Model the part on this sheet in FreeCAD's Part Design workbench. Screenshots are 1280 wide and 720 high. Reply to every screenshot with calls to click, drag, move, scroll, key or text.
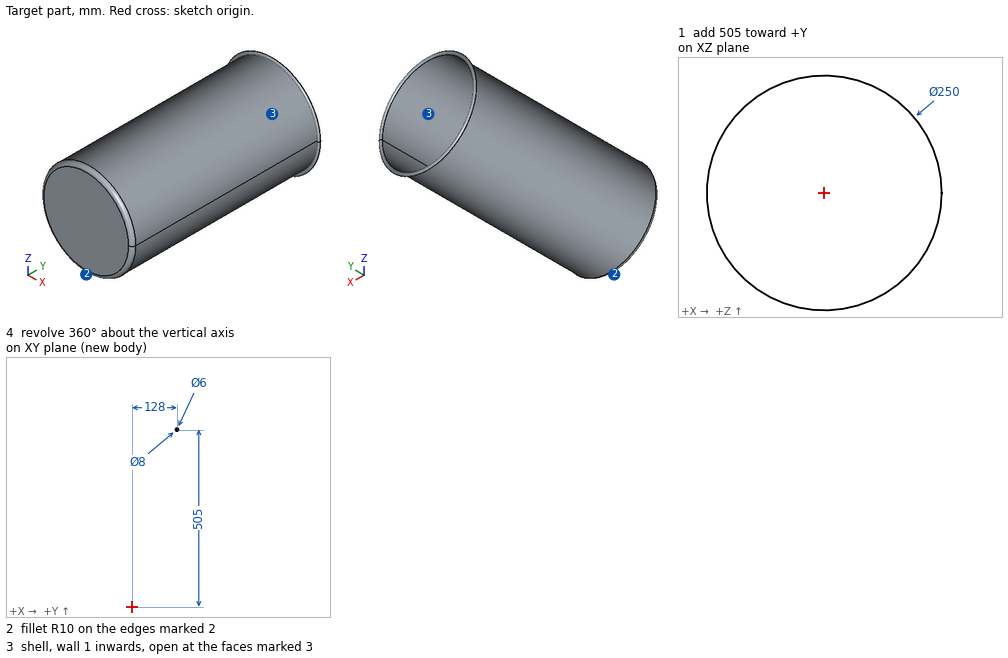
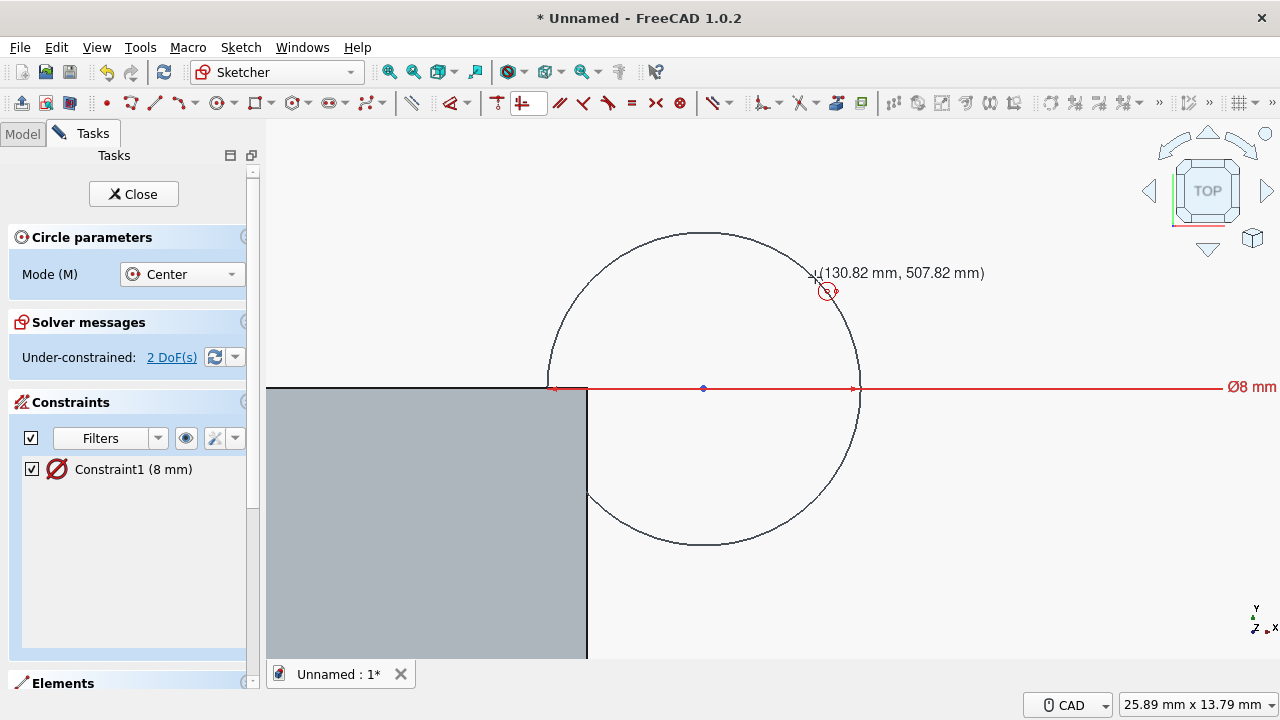
click(704, 389)
move(788, 305)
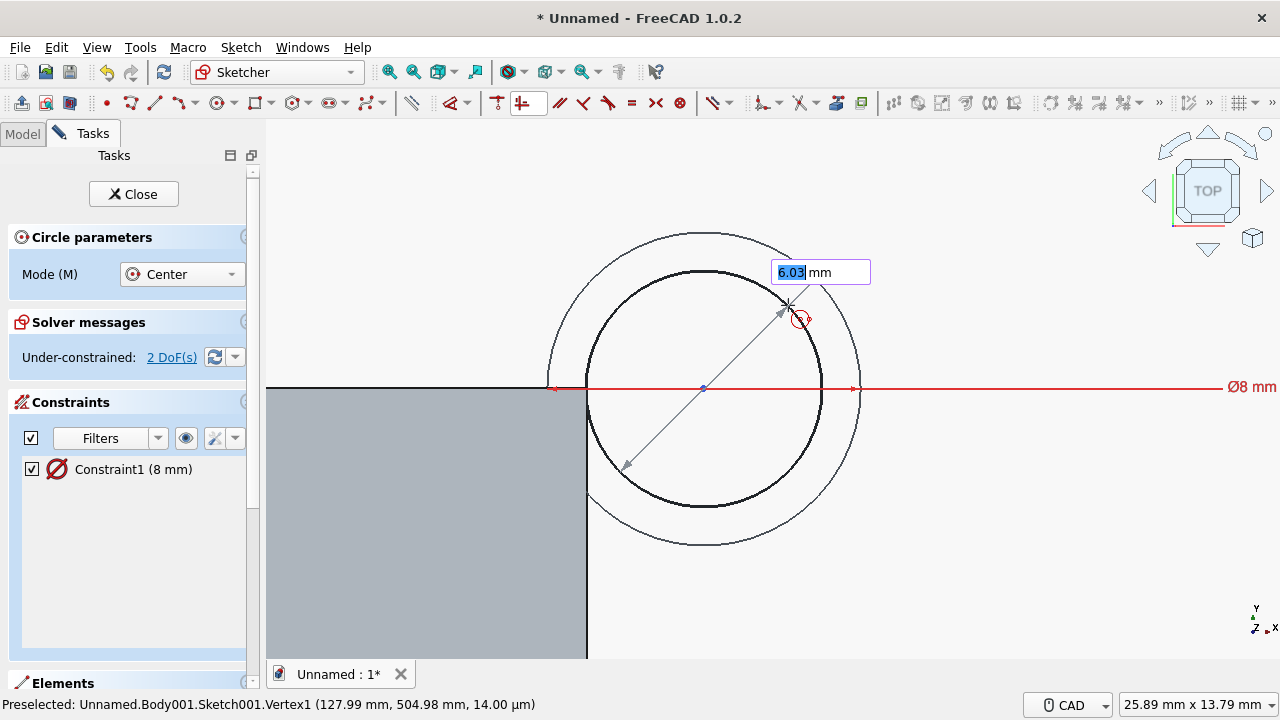
text(6)
key(Return)
key(Escape)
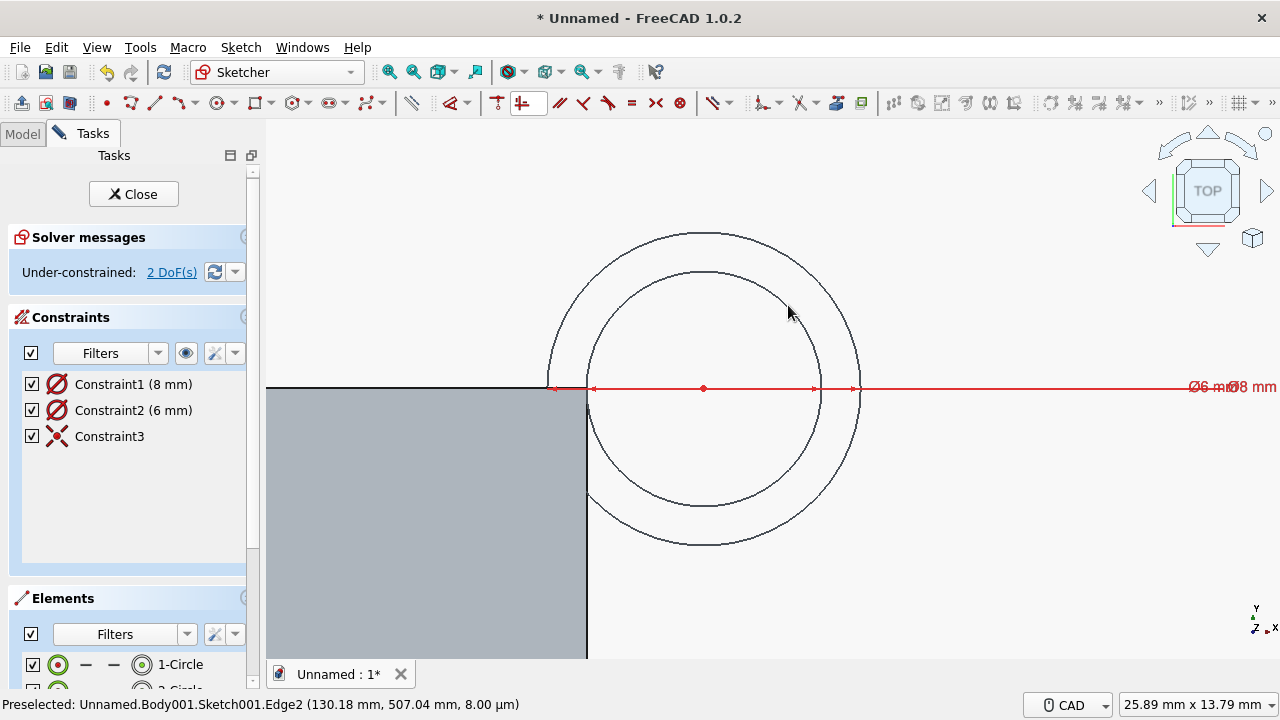
key(d)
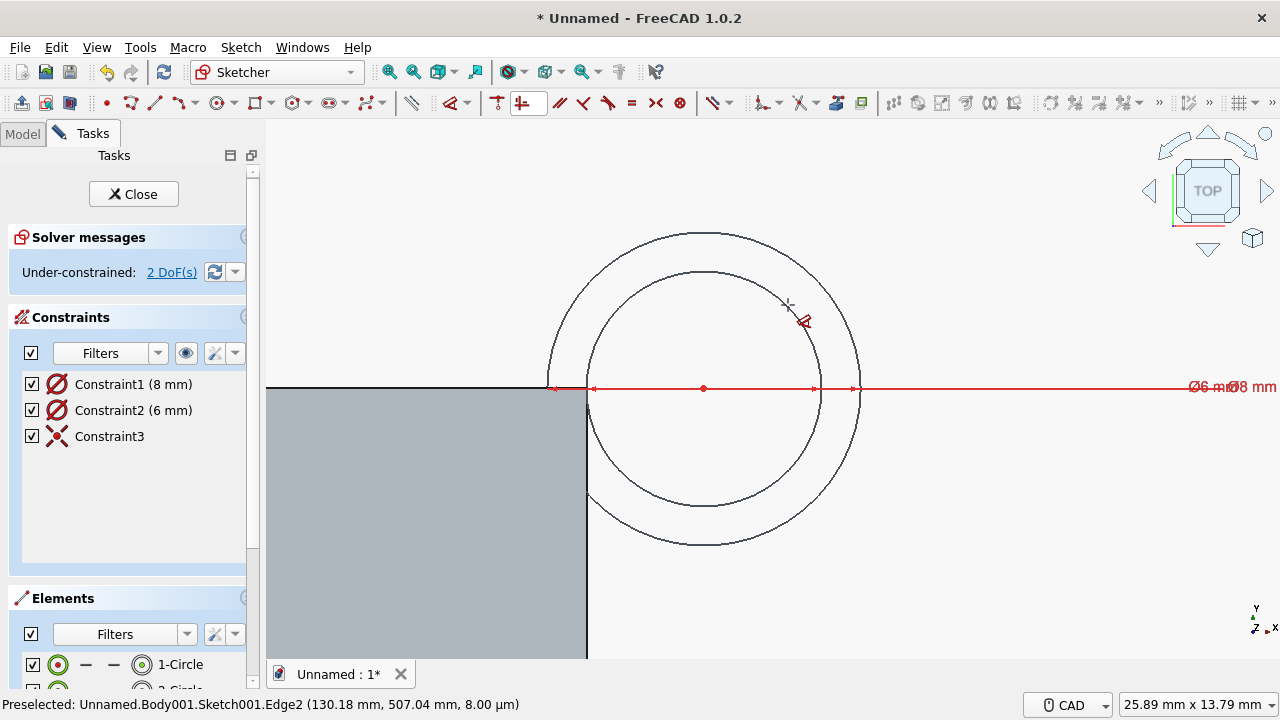
click(704, 389)
click(499, 355)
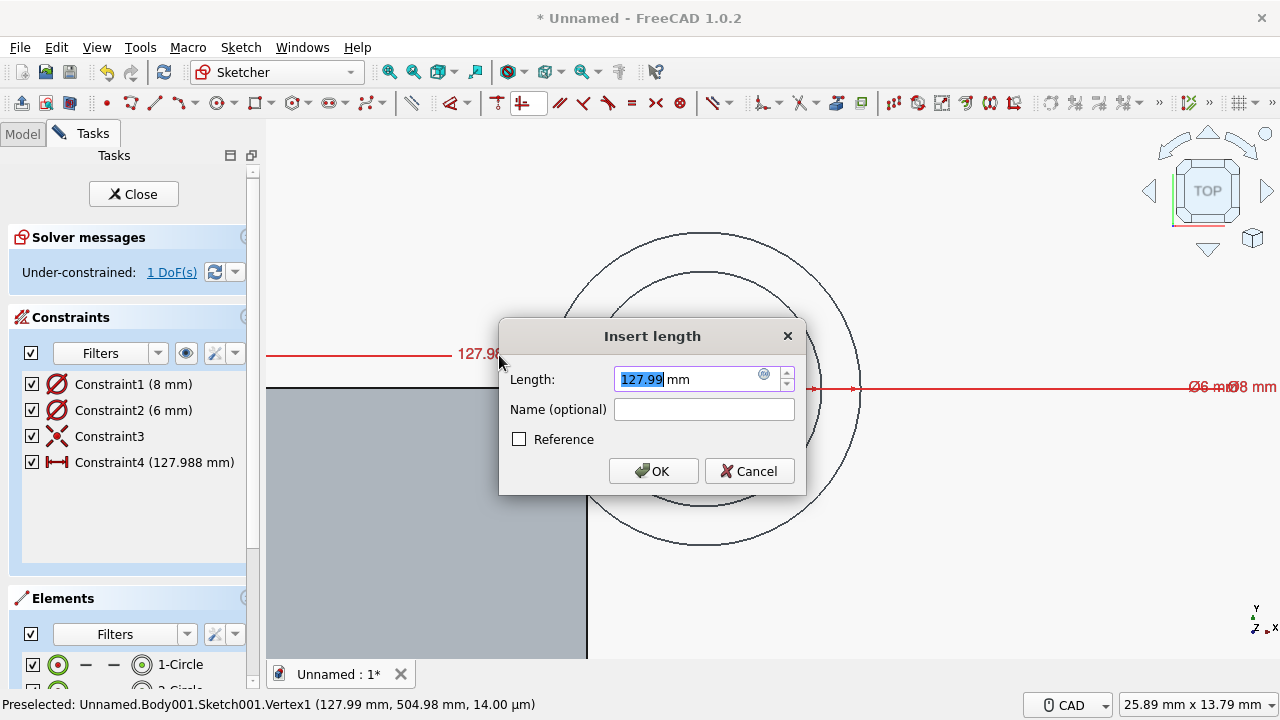
text(128)
key(Return)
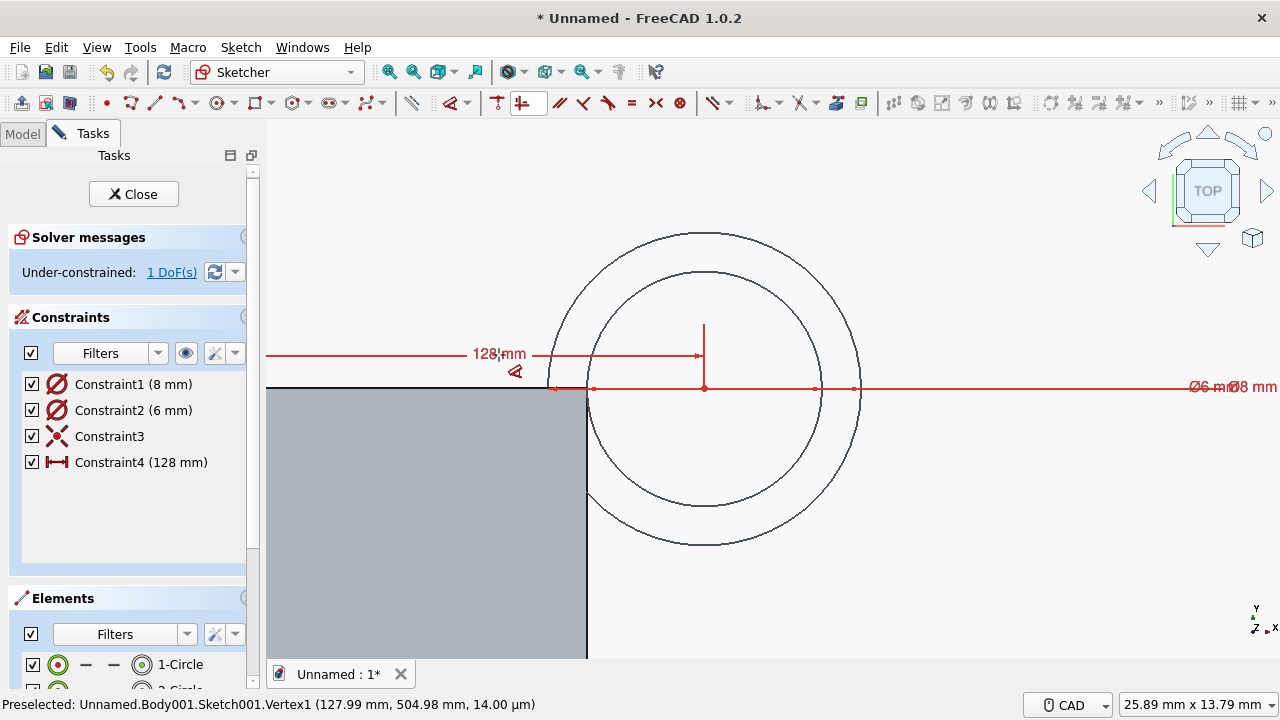
click(704, 389)
click(738, 454)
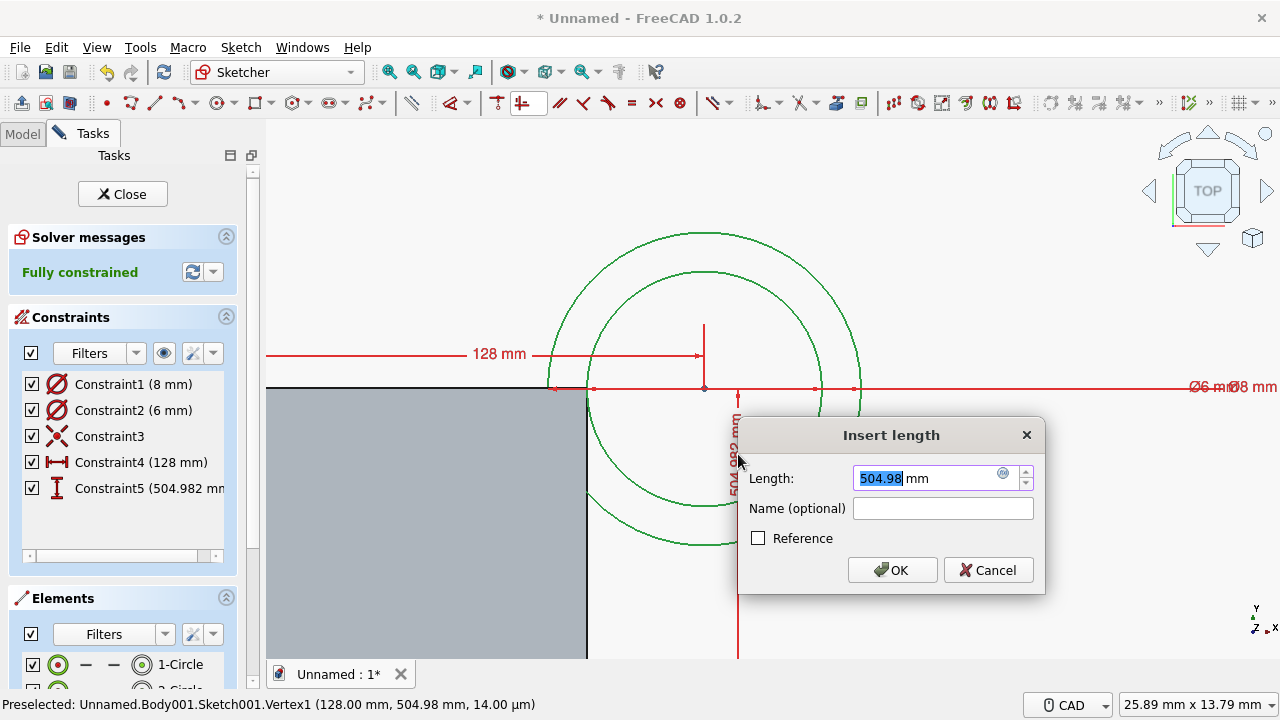
text(505)
key(Return)
key(Escape)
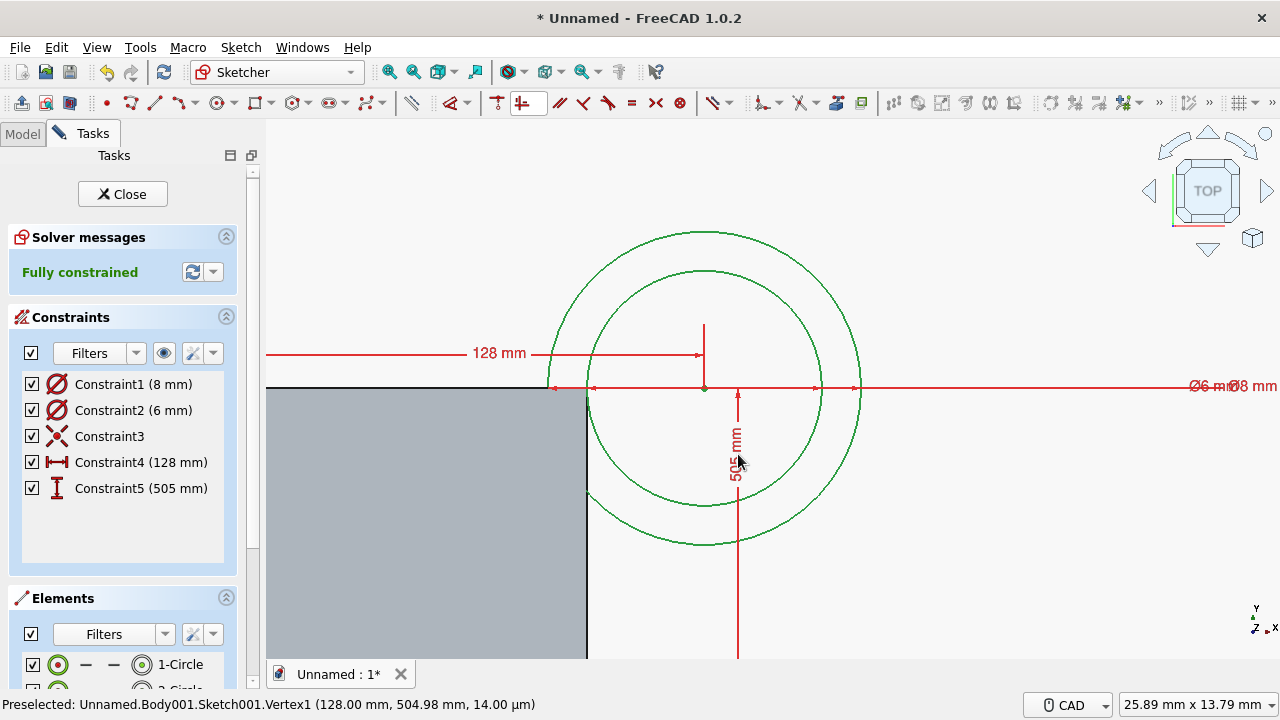
click(123, 194)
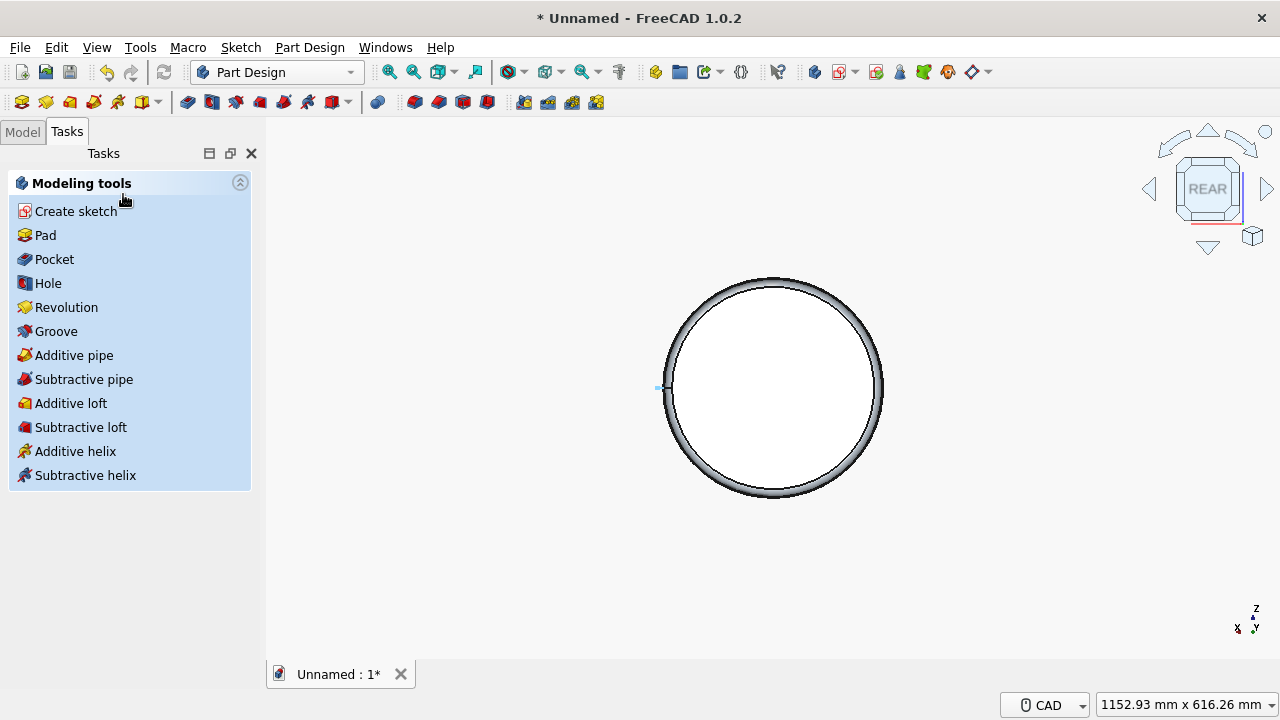
click(46, 102)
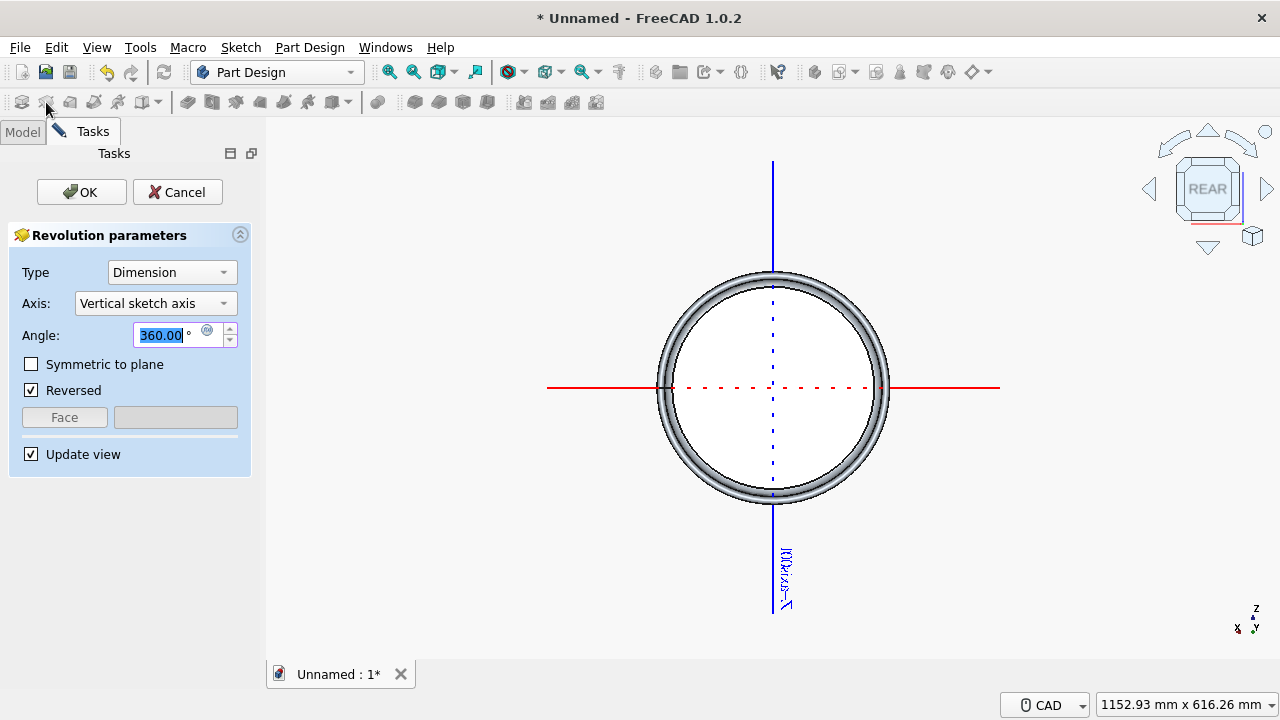
click(82, 192)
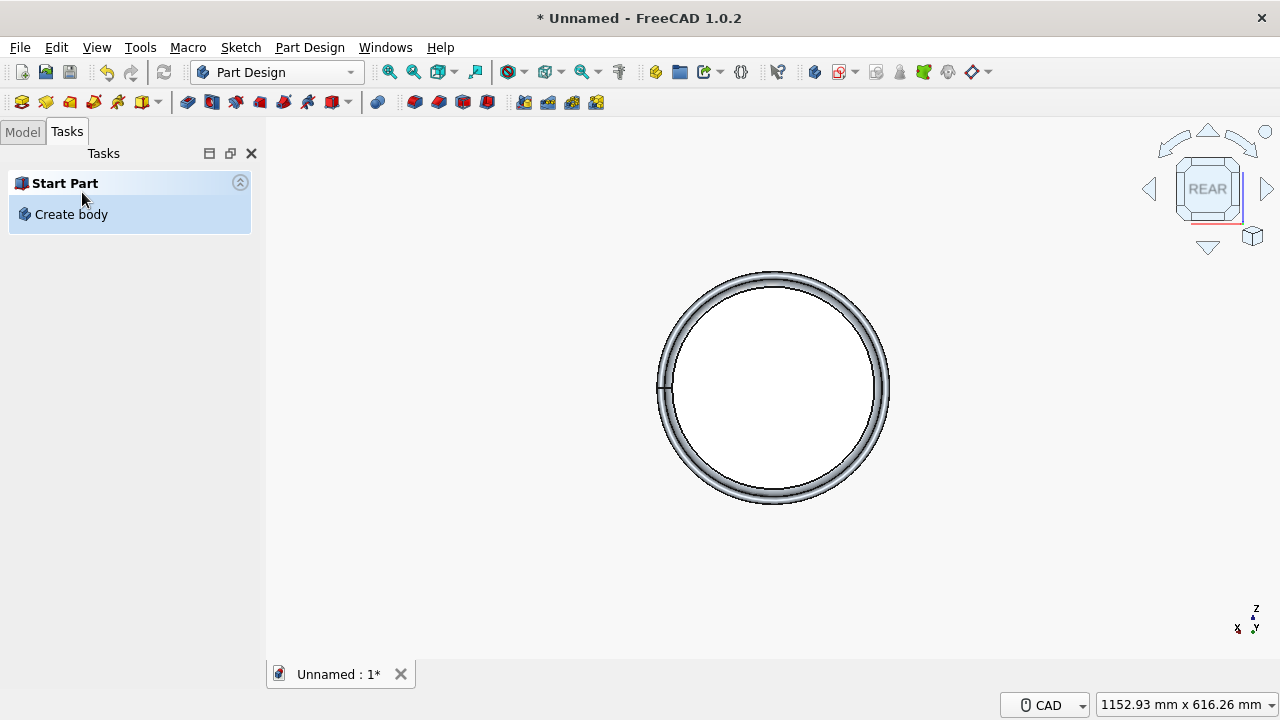
key(0)